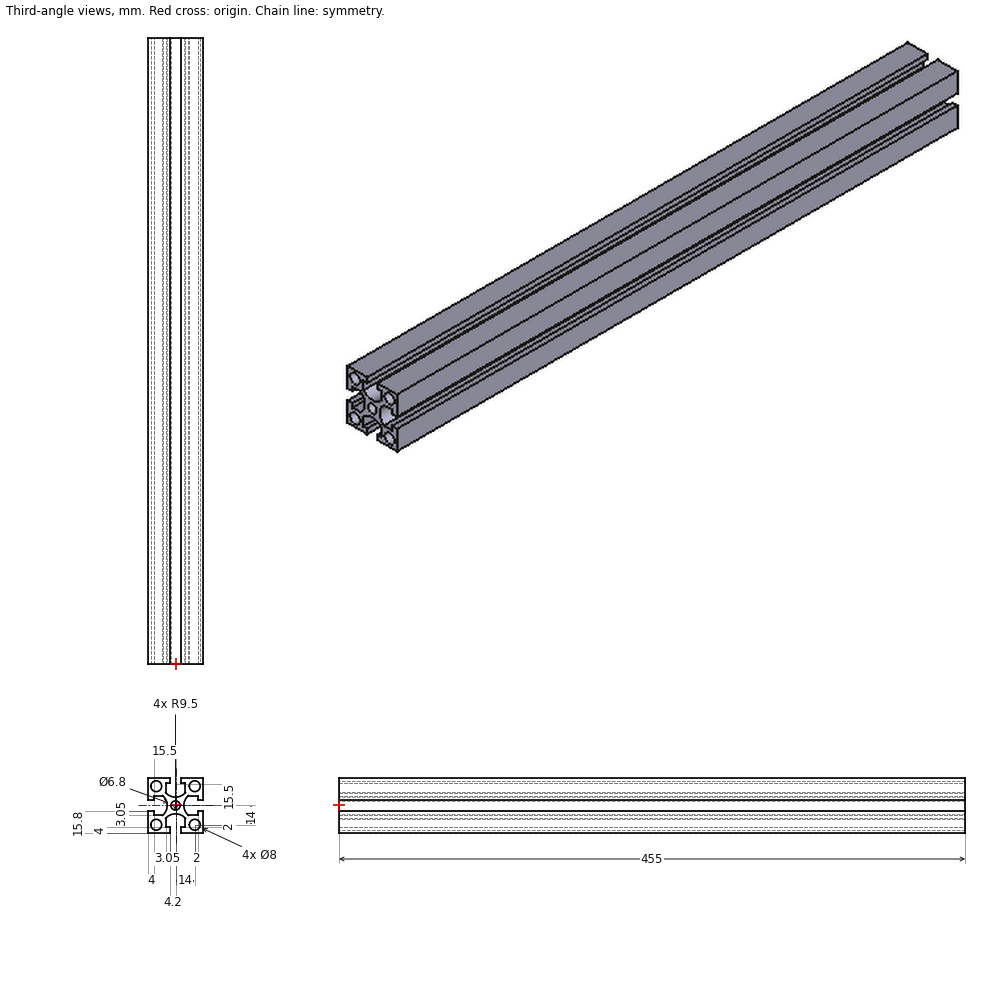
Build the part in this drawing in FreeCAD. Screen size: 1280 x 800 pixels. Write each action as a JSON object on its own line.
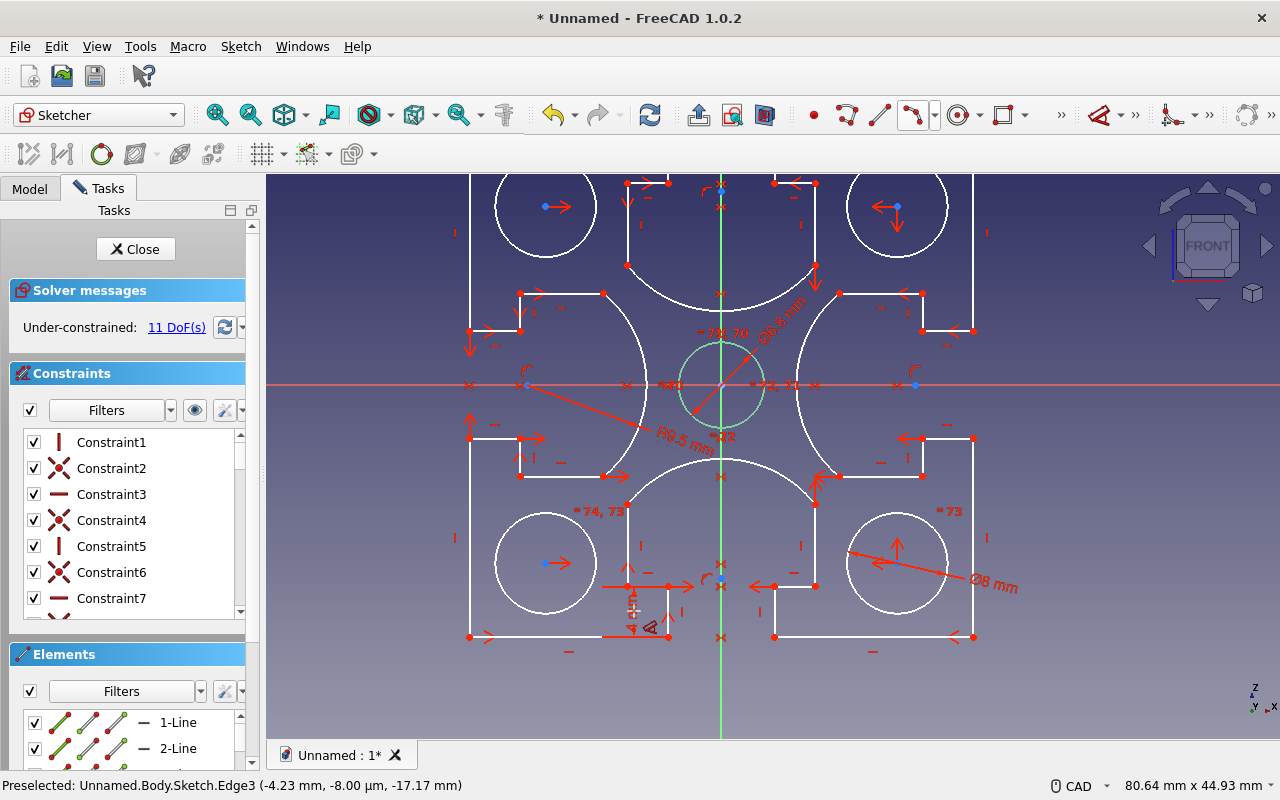
{"action": "left_click", "coordinate": [485, 439]}
{"action": "left_click", "coordinate": [495, 473]}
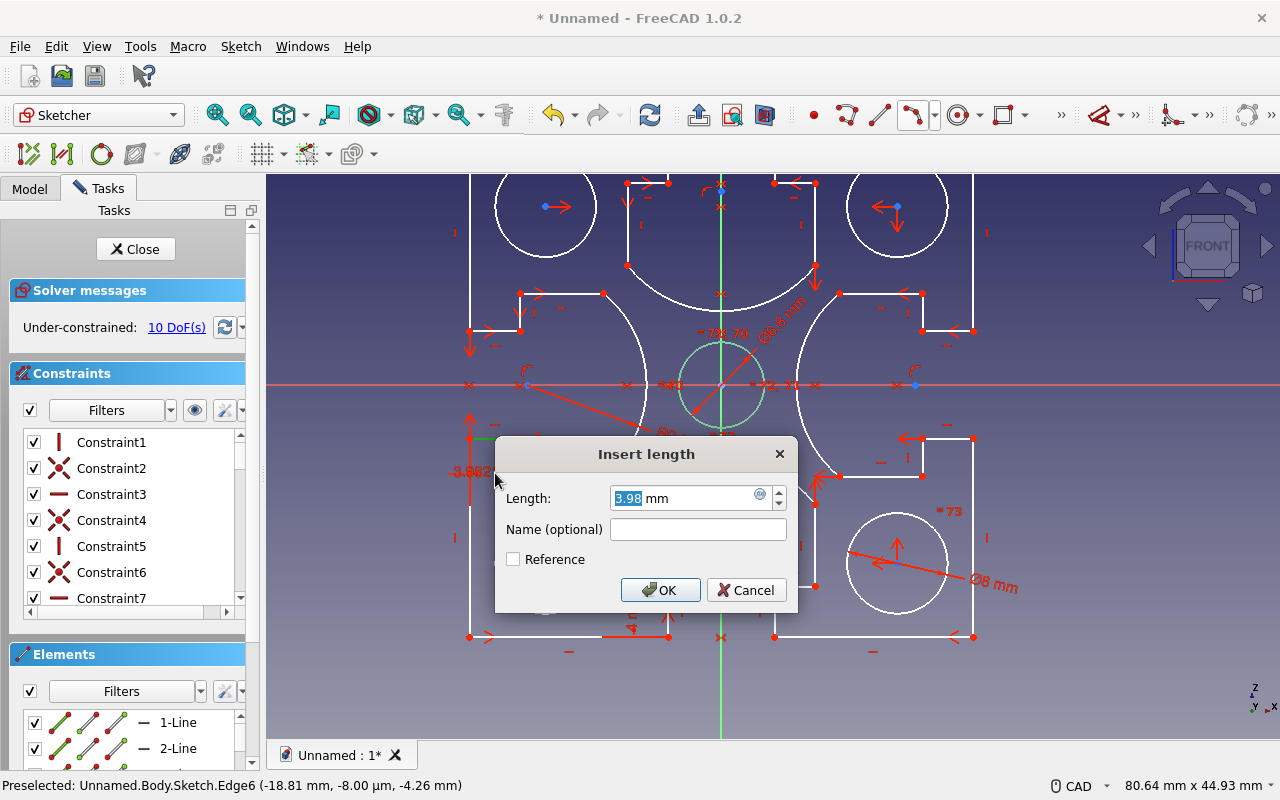
{"action": "type", "text": "4"}
{"action": "key", "text": "Return"}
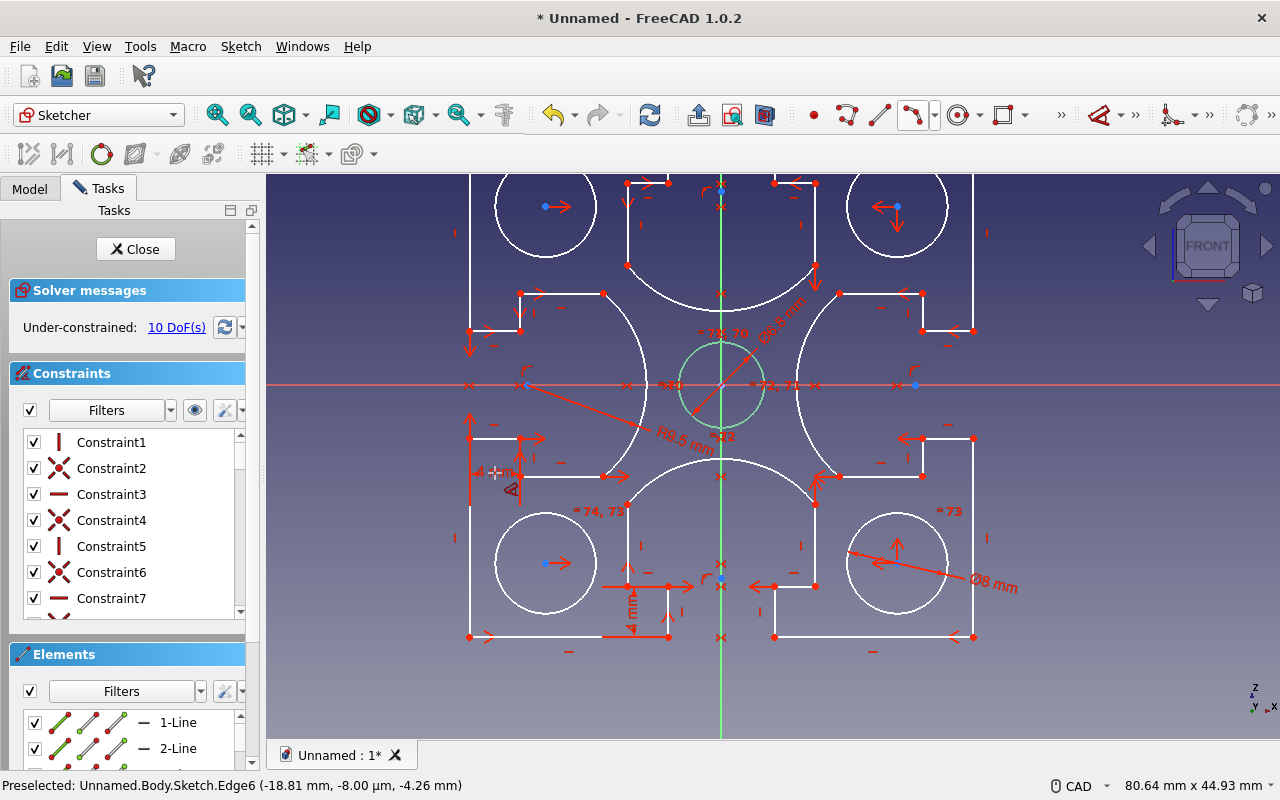
{"action": "left_click", "coordinate": [897, 563]}
{"action": "left_click", "coordinate": [748, 597]}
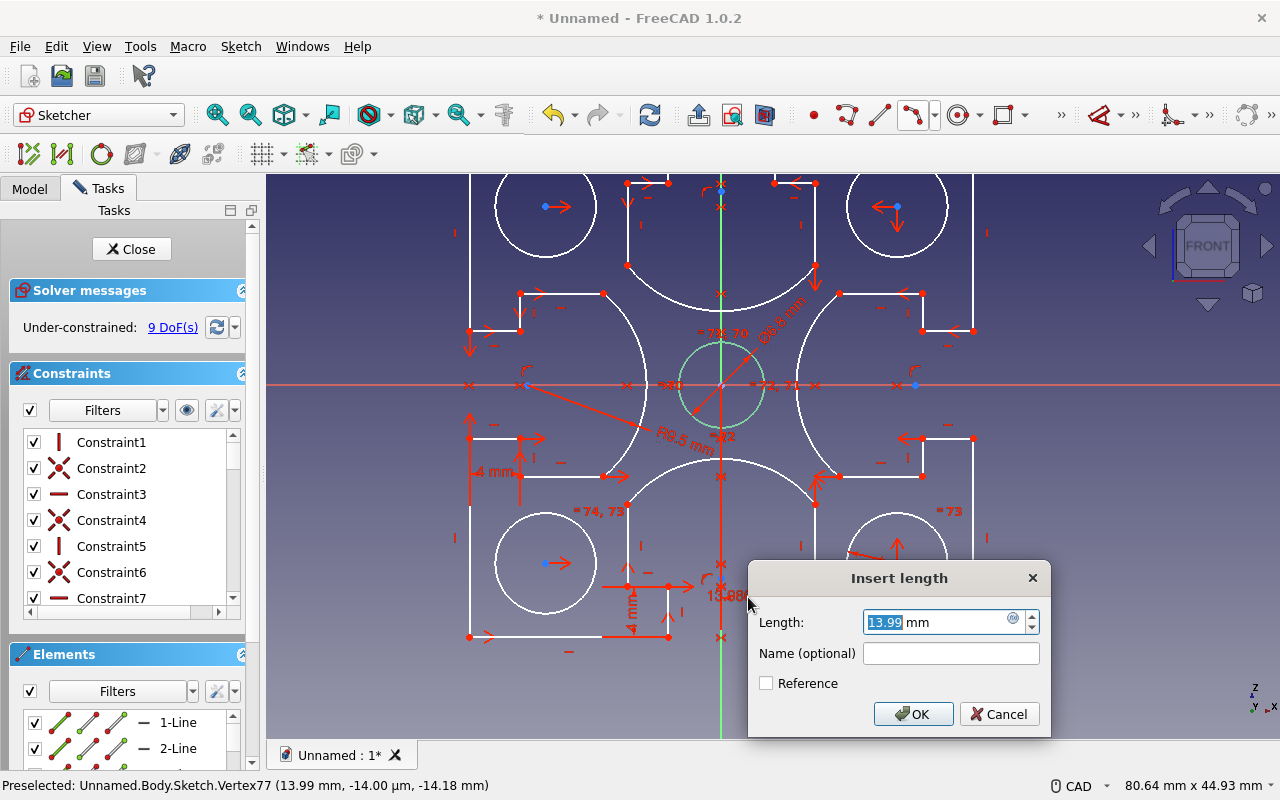
{"action": "type", "text": "14"}
{"action": "key", "text": "Return"}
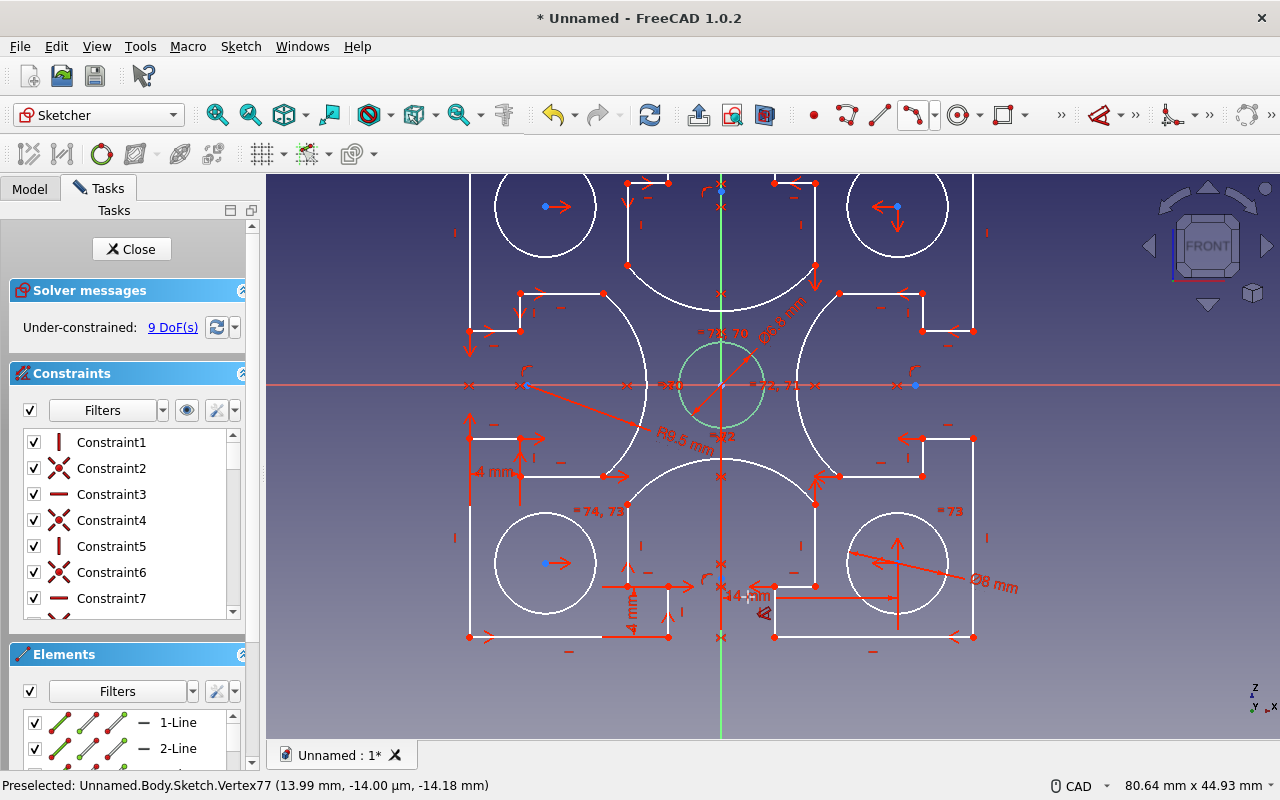
{"action": "left_click", "coordinate": [898, 563]}
{"action": "left_click", "coordinate": [932, 412]}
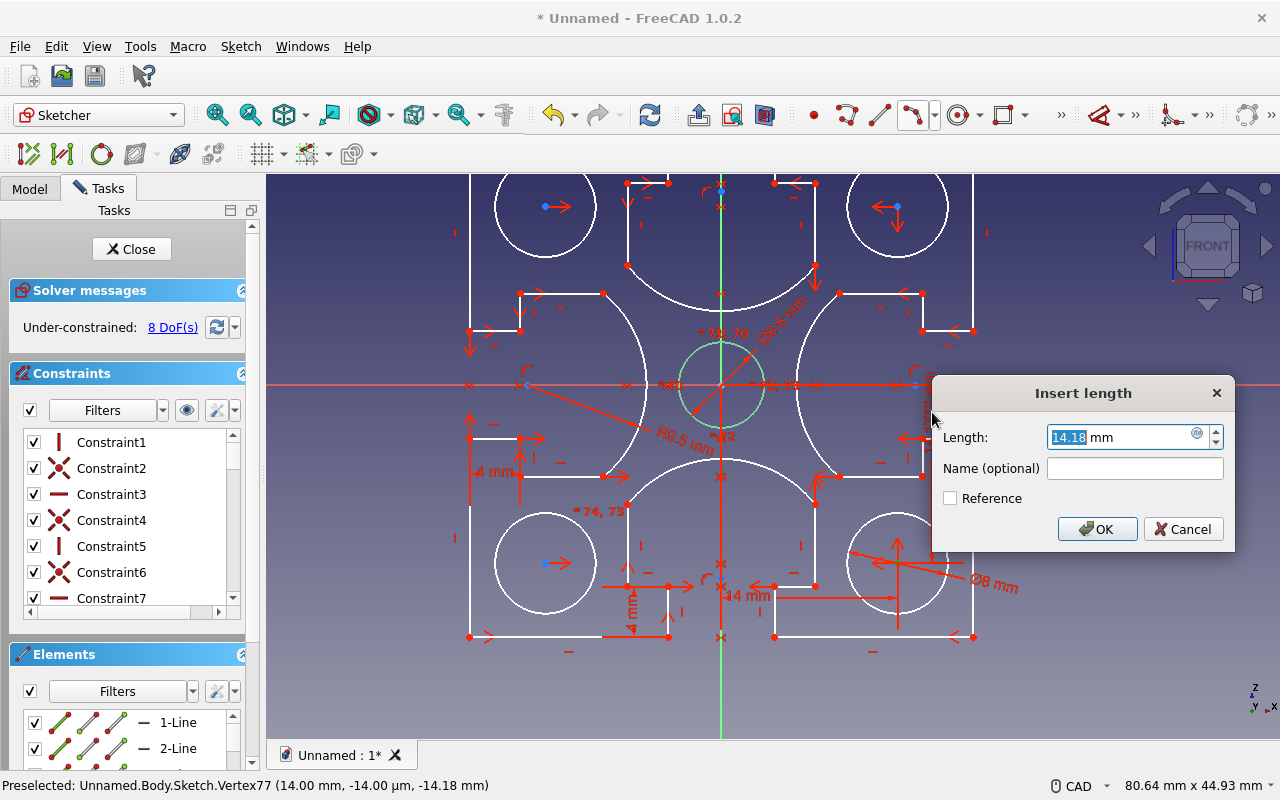
{"action": "type", "text": "14"}
{"action": "key", "text": "Return"}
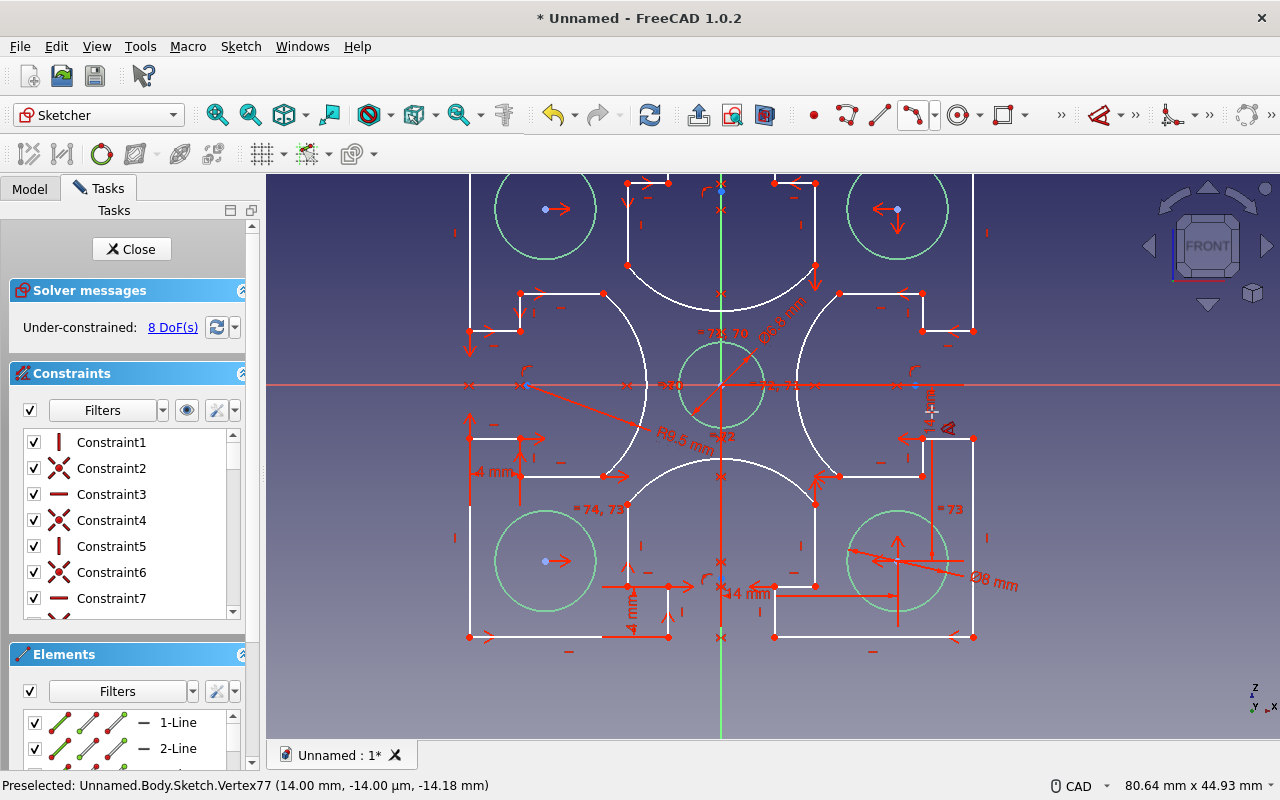
{"action": "scroll", "coordinate": [923, 477], "scroll_direction": "up", "scroll_amount": 3}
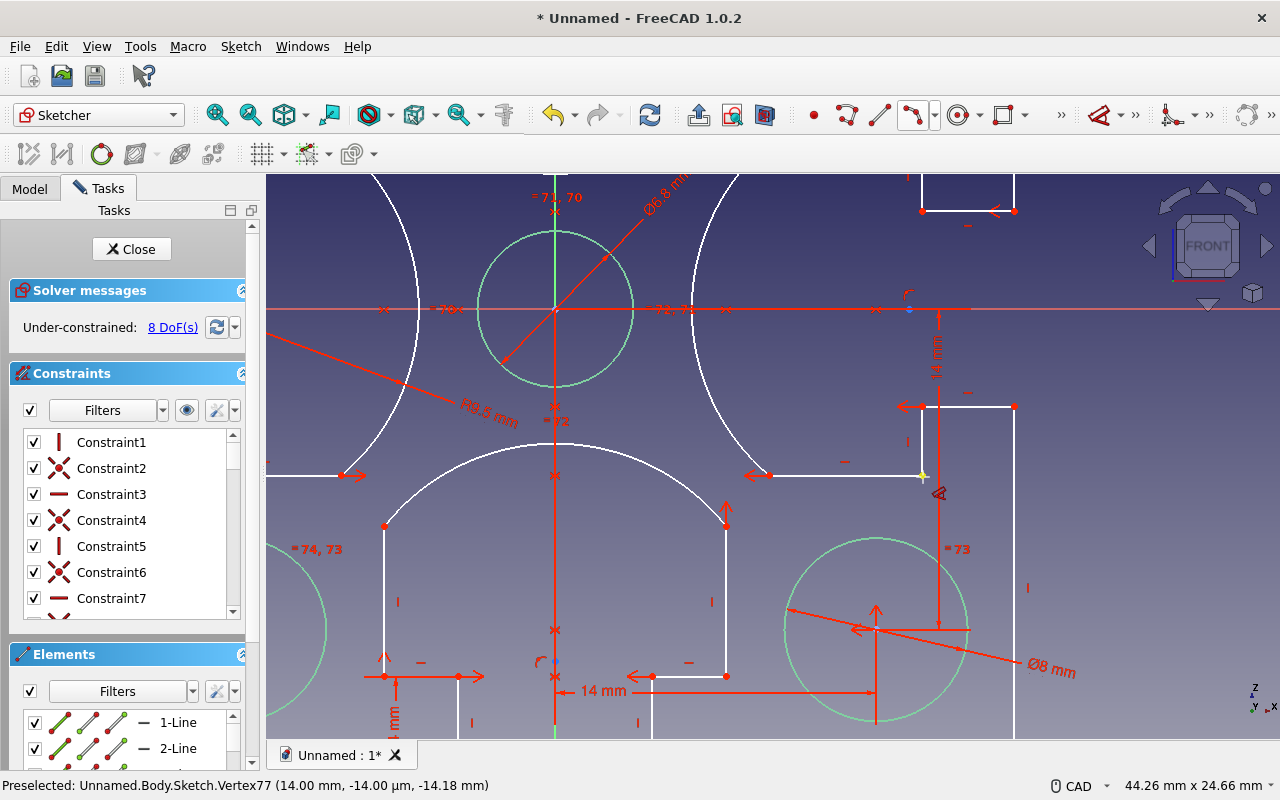
{"action": "left_click", "coordinate": [922, 476]}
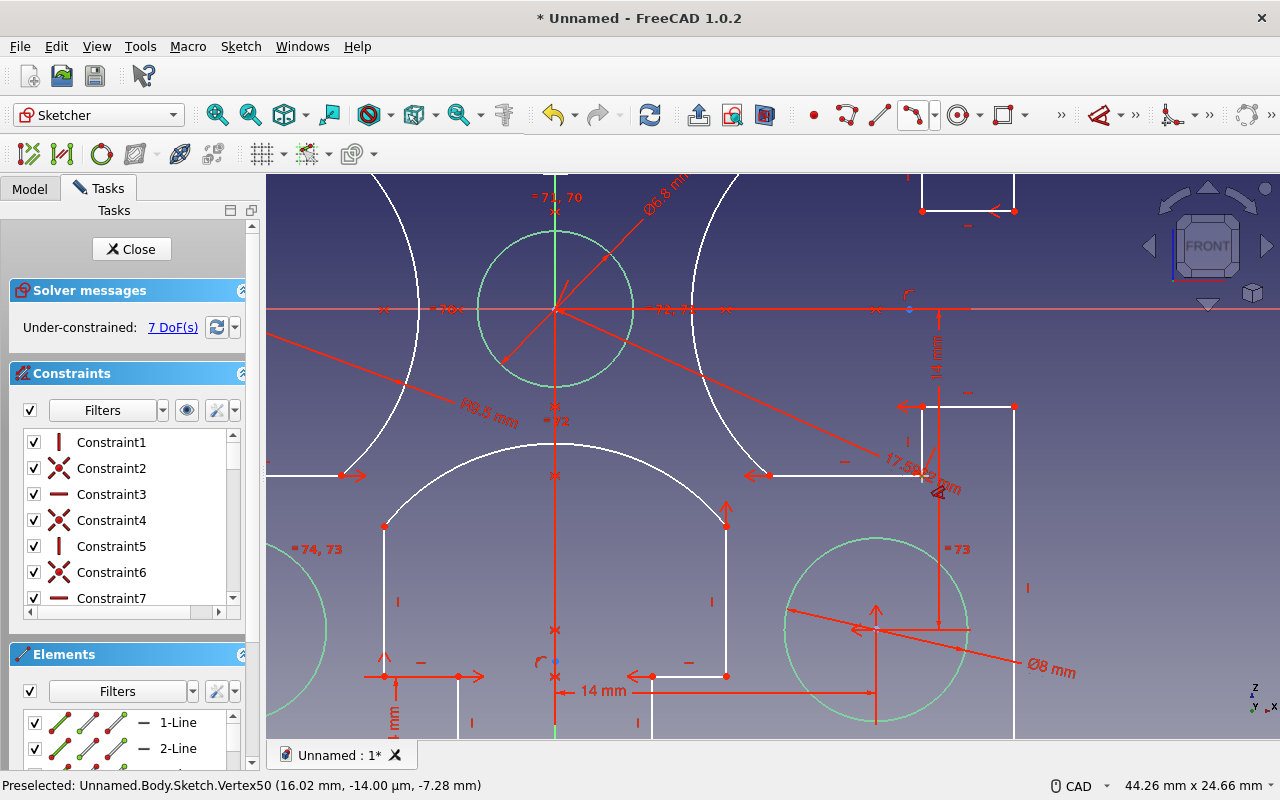
{"action": "left_click", "coordinate": [876, 630]}
{"action": "left_click", "coordinate": [899, 664]}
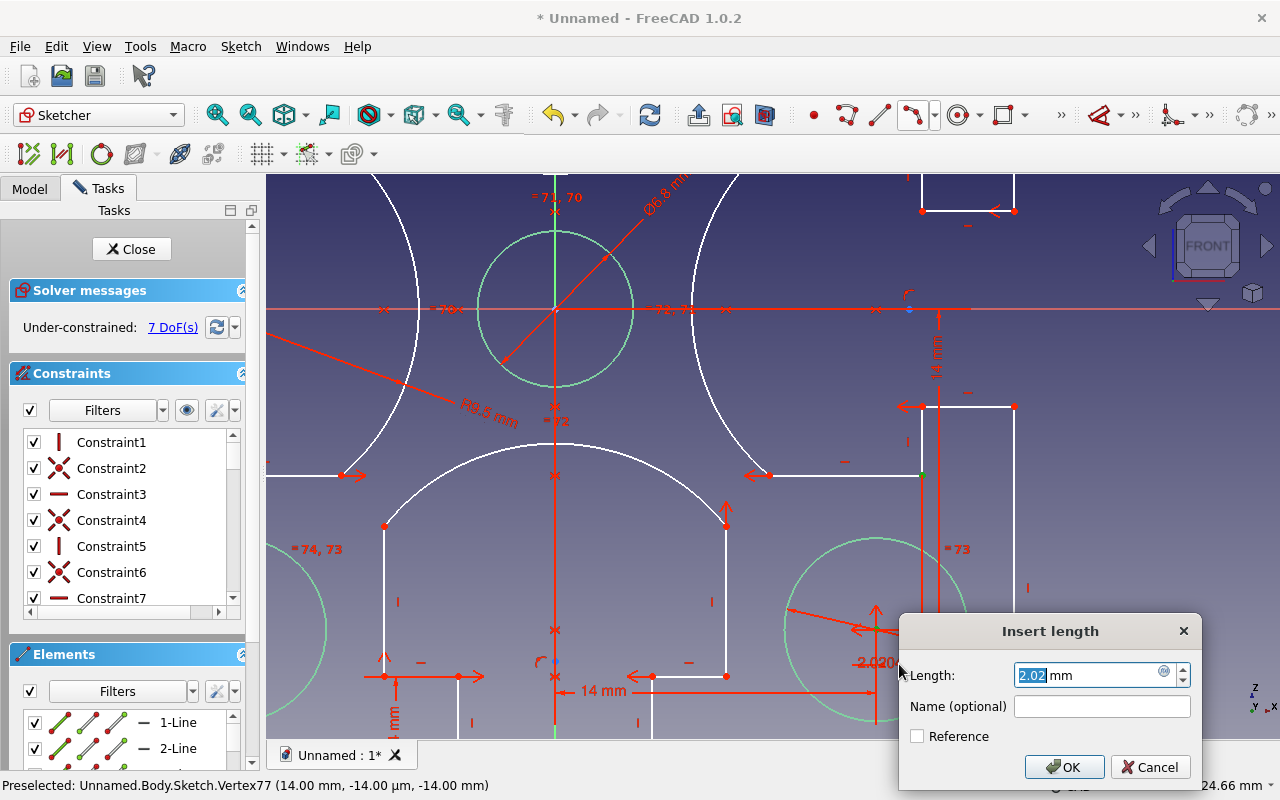
{"action": "type", "text": "2"}
{"action": "key", "text": "Return"}